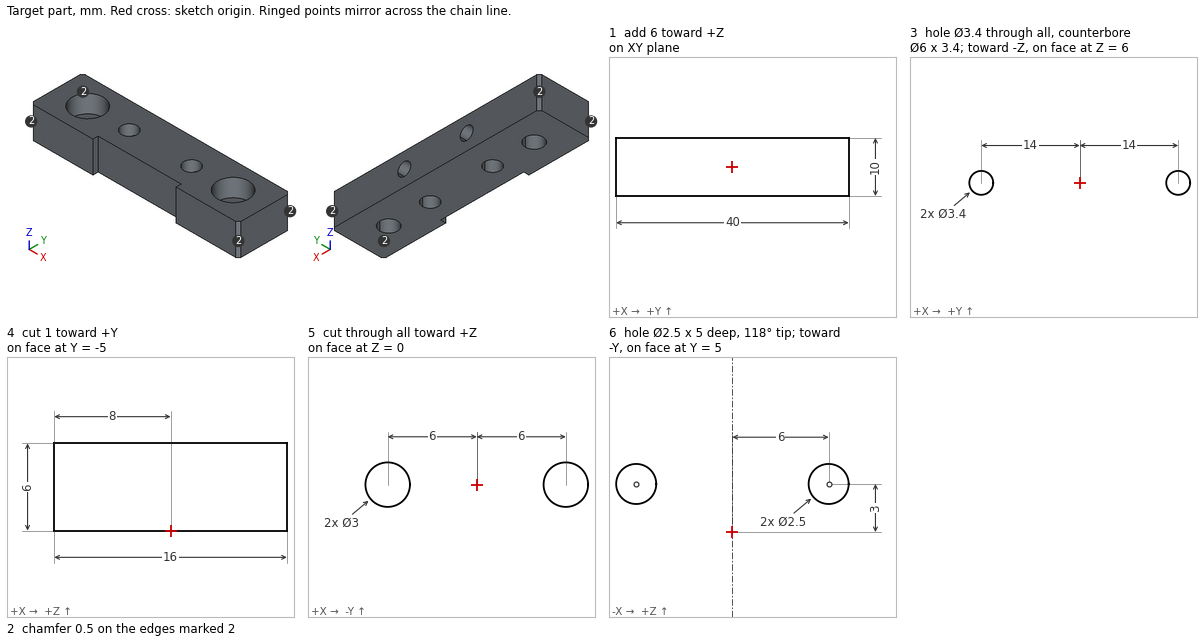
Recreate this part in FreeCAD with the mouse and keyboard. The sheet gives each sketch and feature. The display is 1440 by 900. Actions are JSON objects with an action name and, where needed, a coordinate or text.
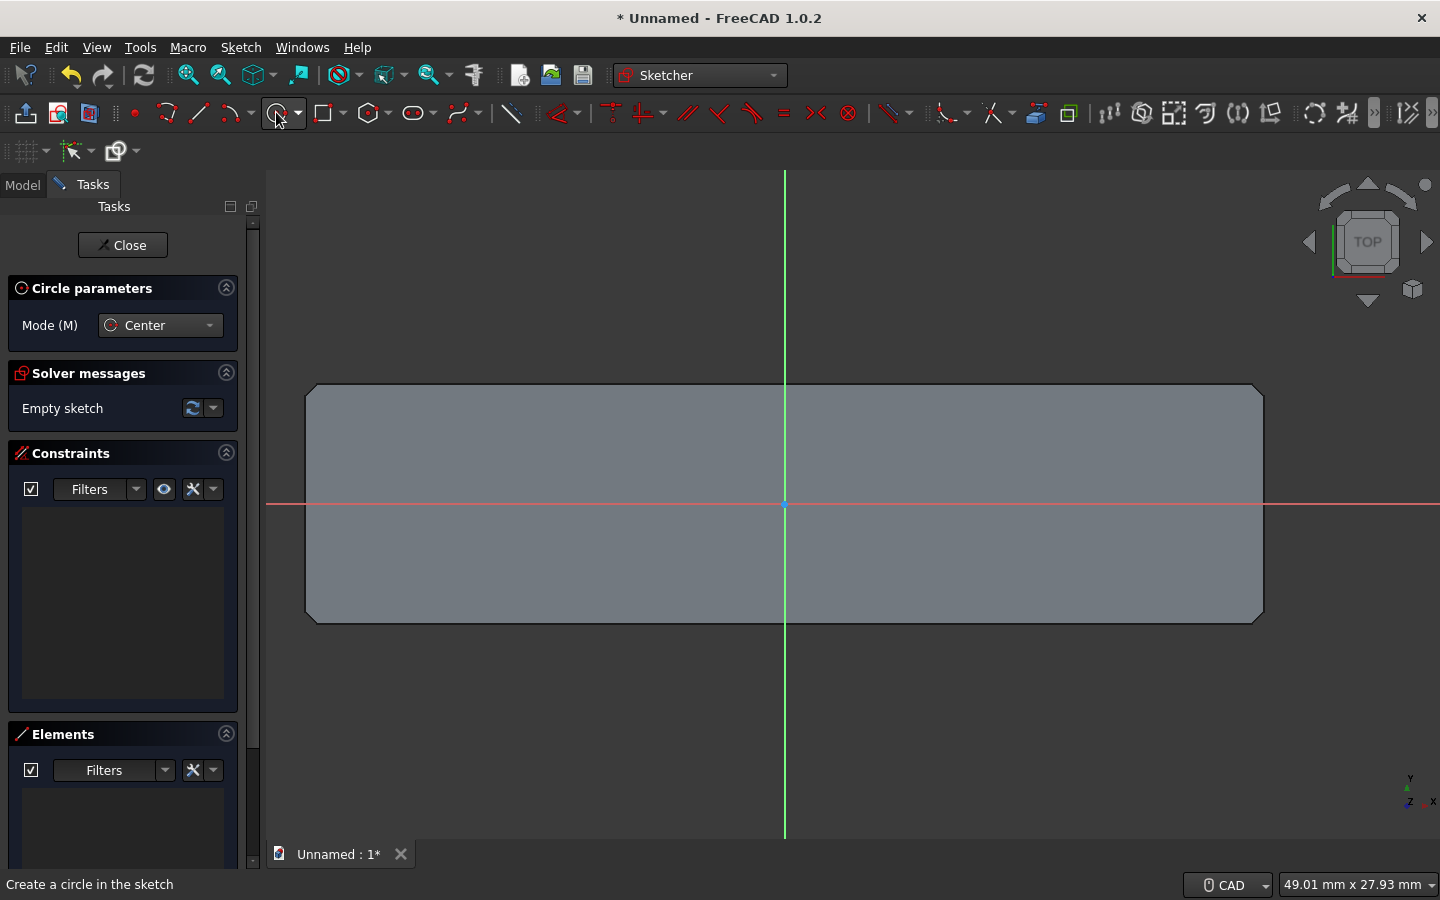
{"action": "left_click", "coordinate": [449, 504]}
{"action": "mouse_move", "coordinate": [478, 475]}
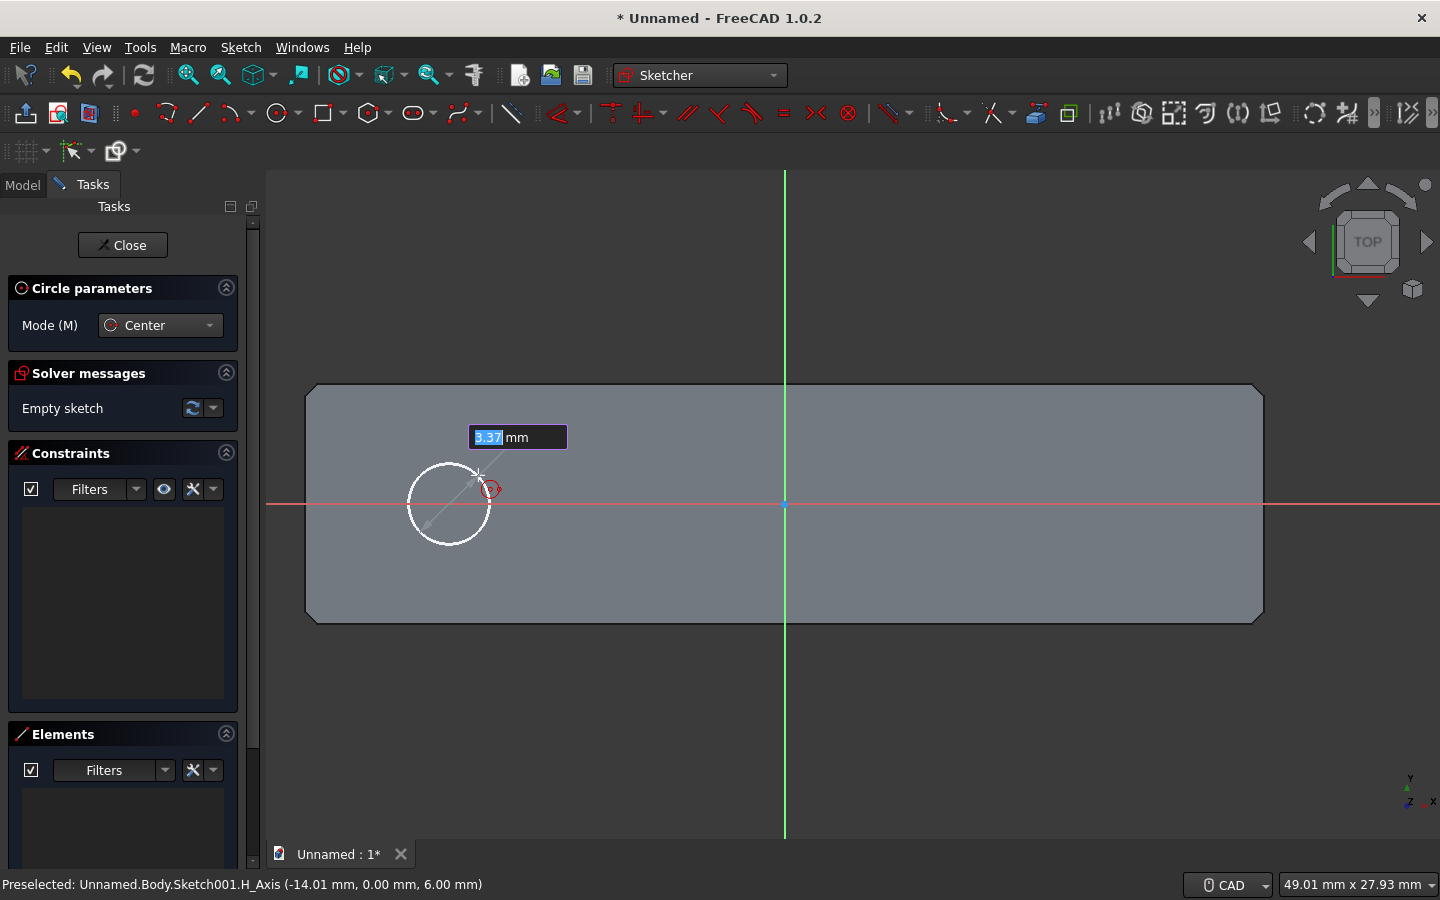
{"action": "type", "text": "3.4"}
{"action": "key", "text": "Return"}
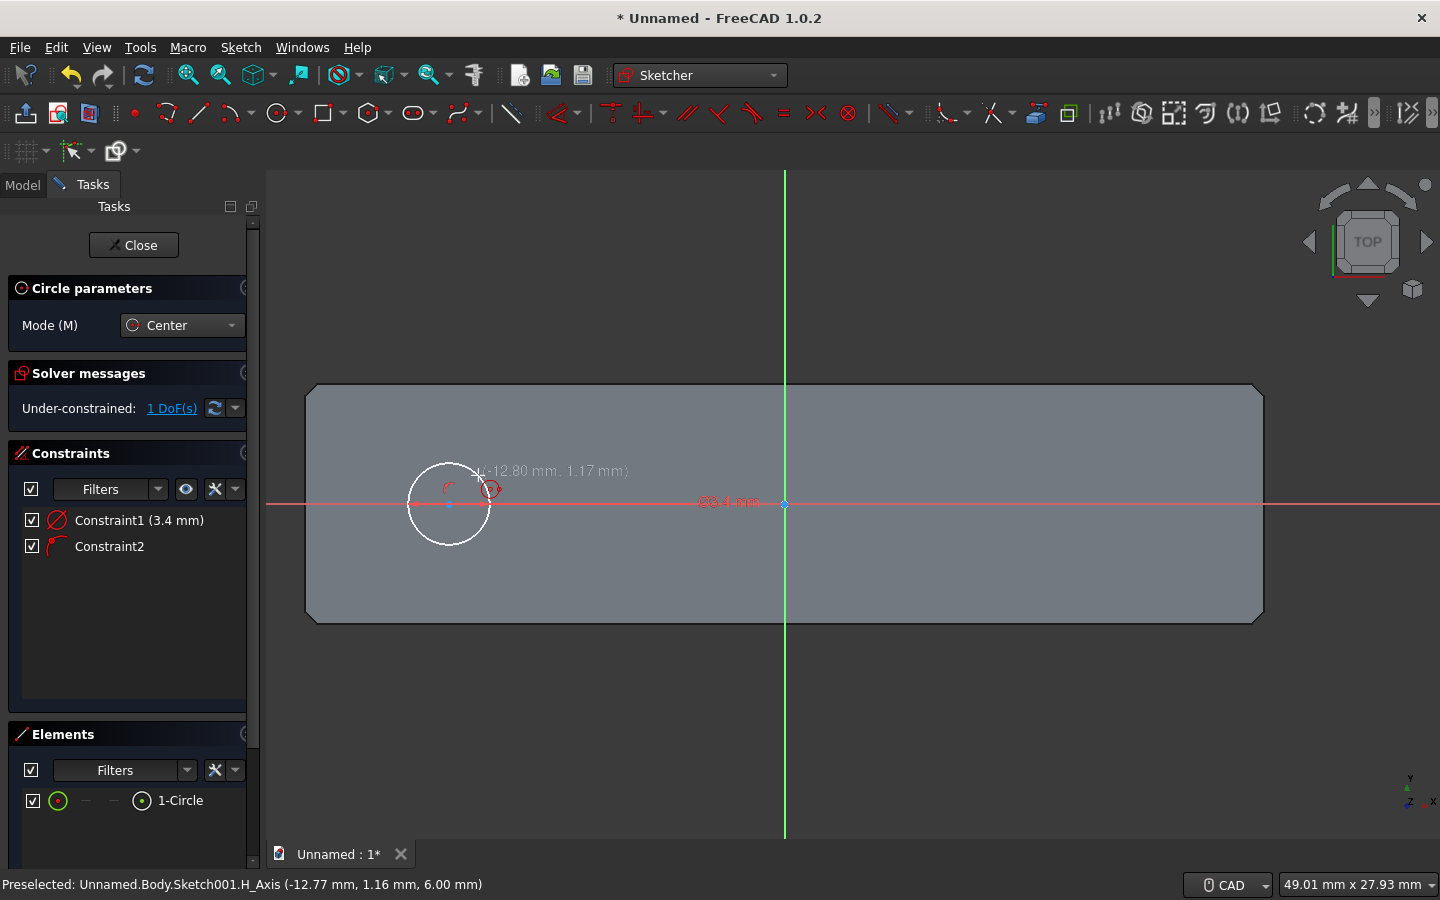
{"action": "left_click", "coordinate": [1120, 504]}
{"action": "mouse_move", "coordinate": [1149, 475]}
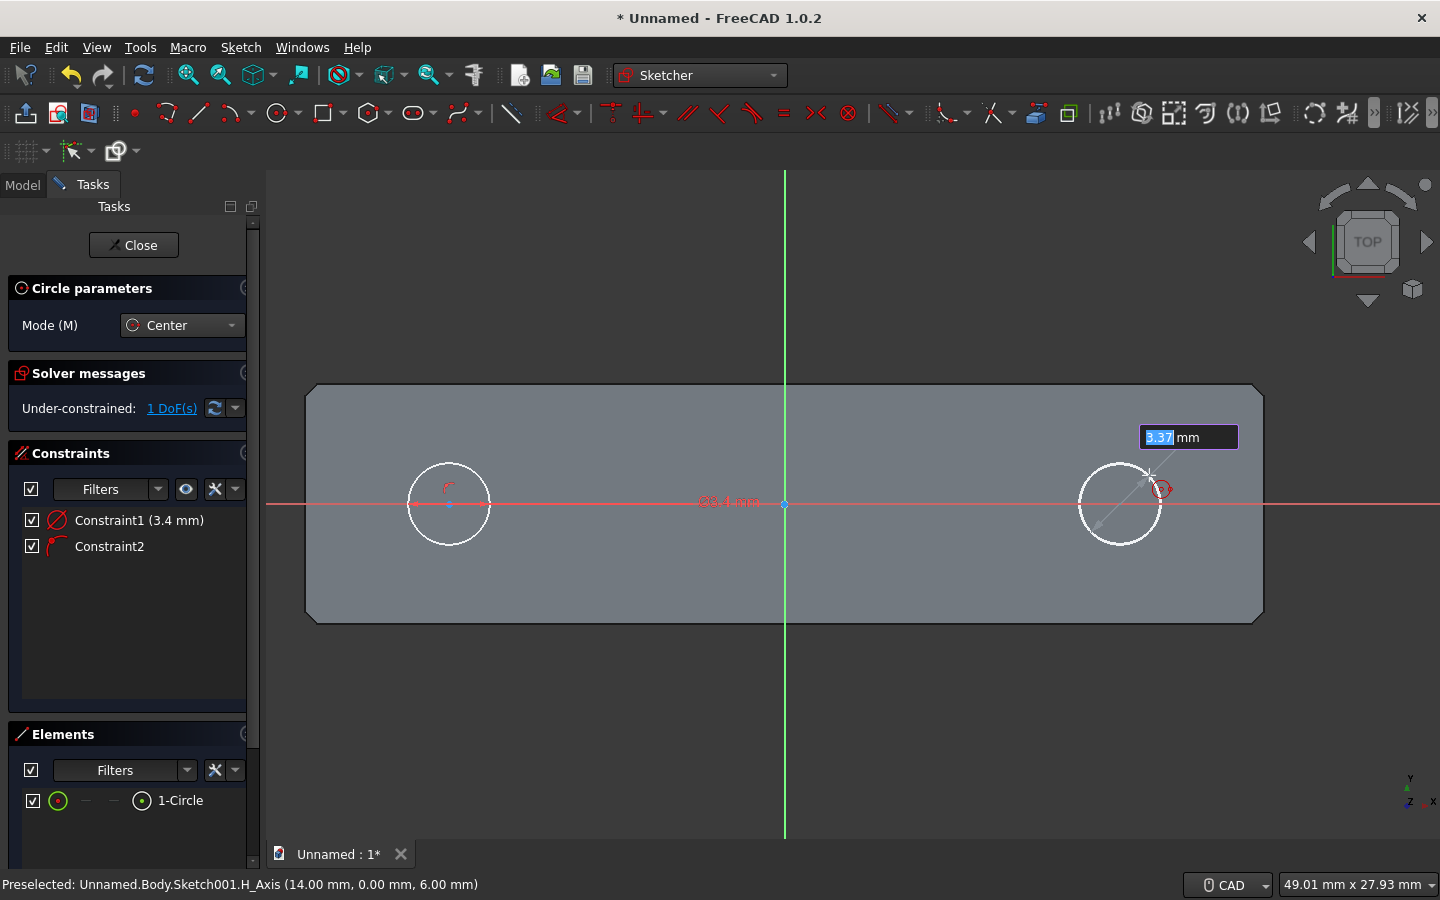
{"action": "type", "text": "3.4"}
{"action": "key", "text": "Return"}
{"action": "key", "text": "Escape"}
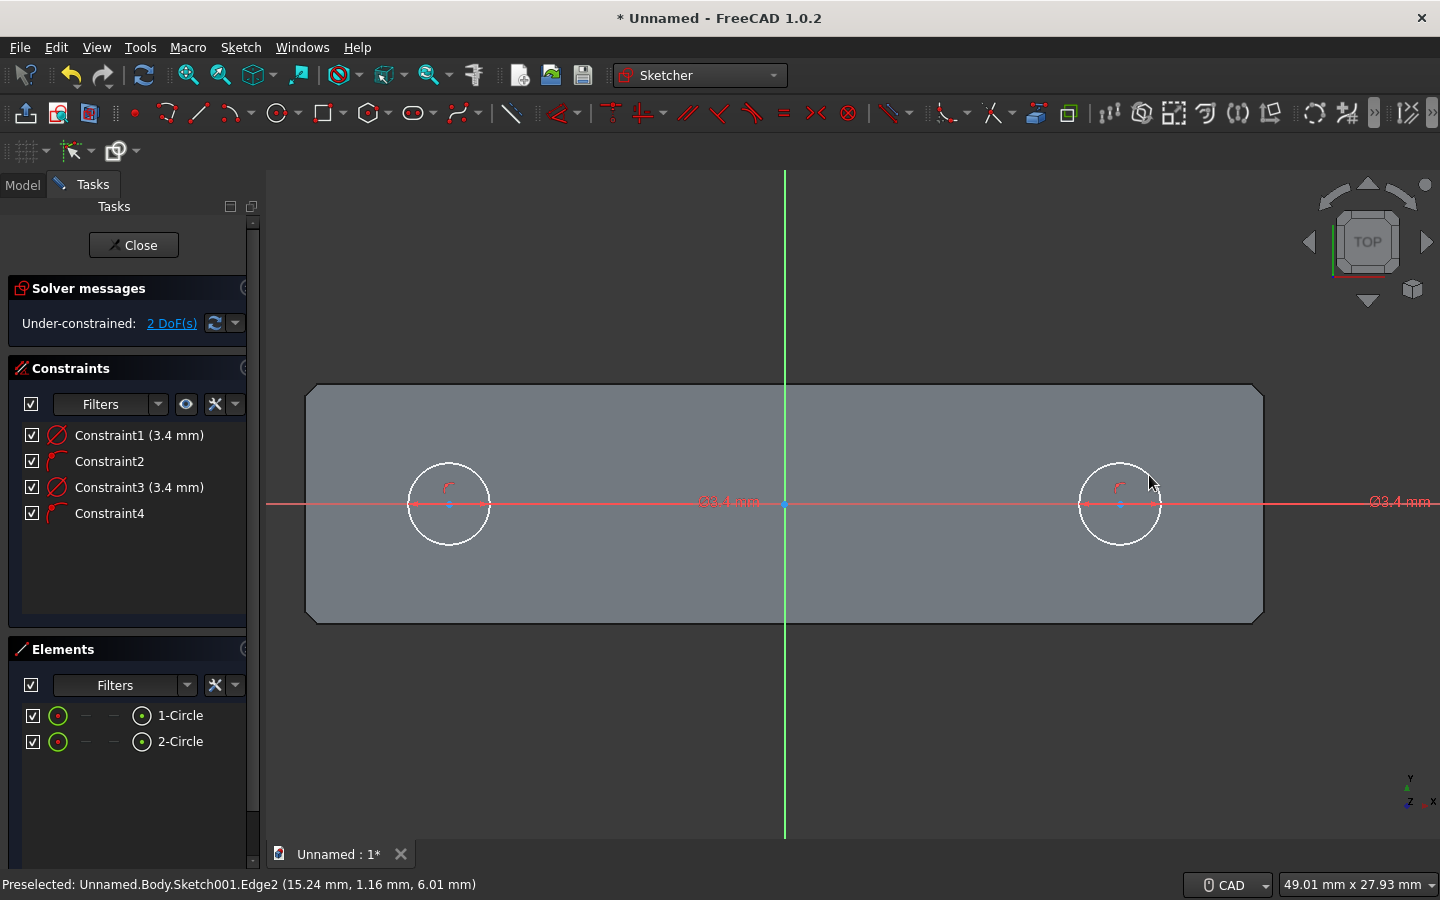
{"action": "left_click", "coordinate": [449, 504]}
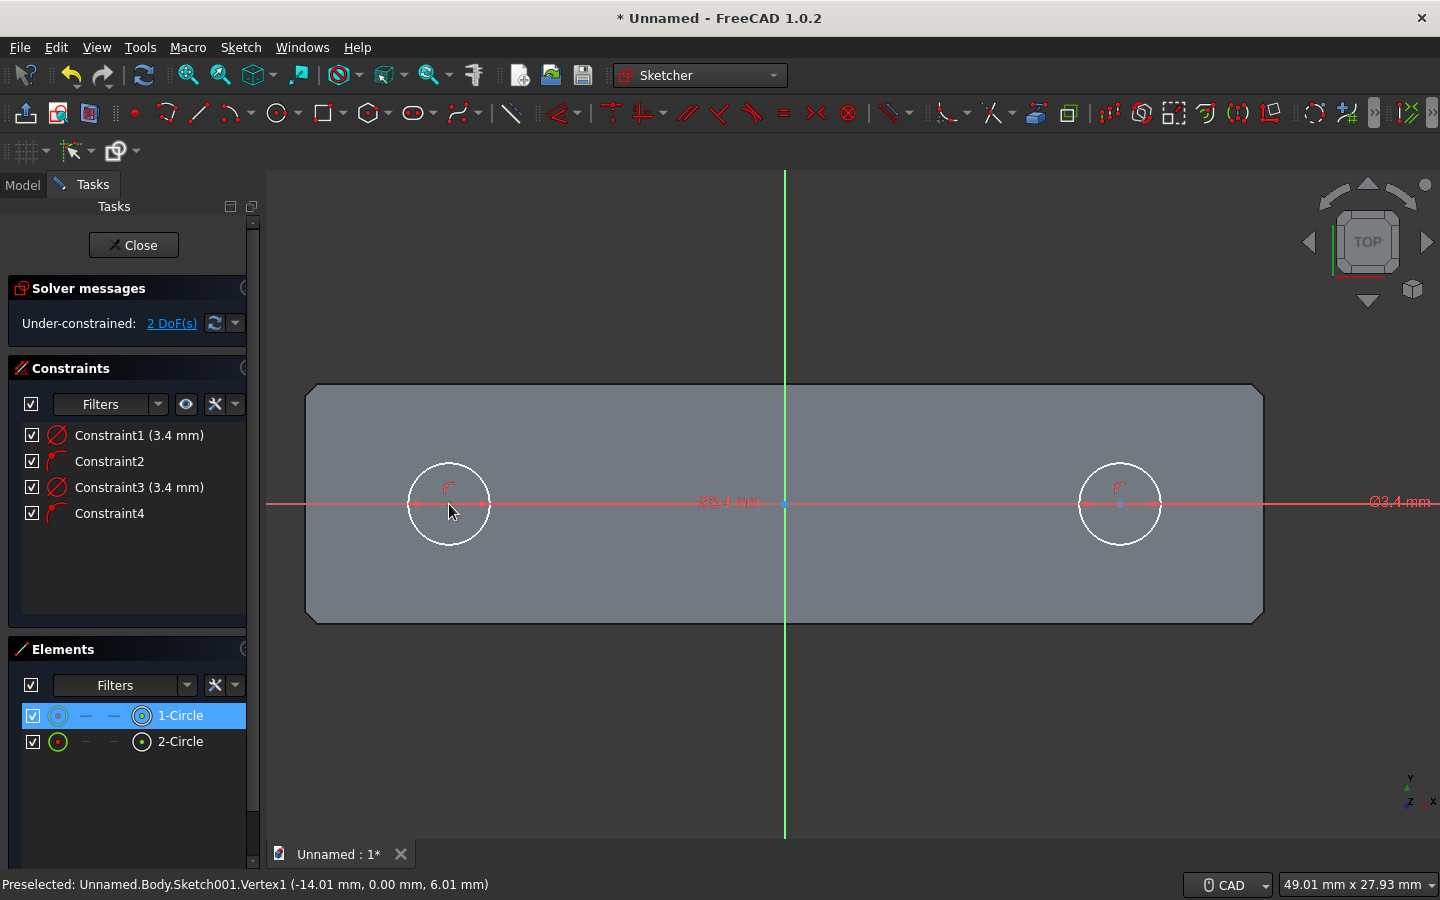
{"action": "left_click", "coordinate": [580, 114]}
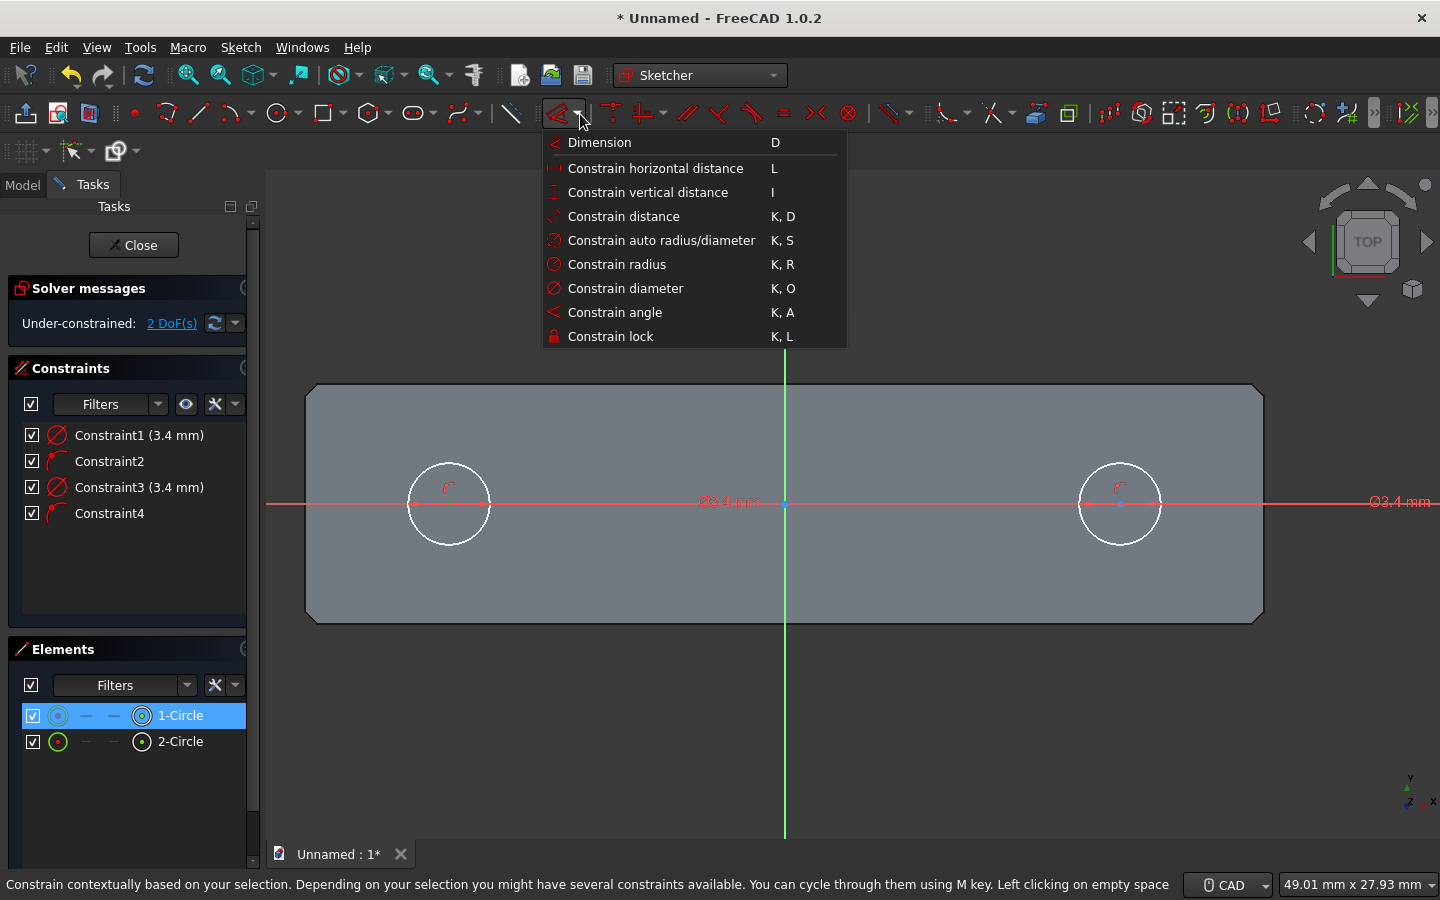
{"action": "left_click", "coordinate": [695, 168]}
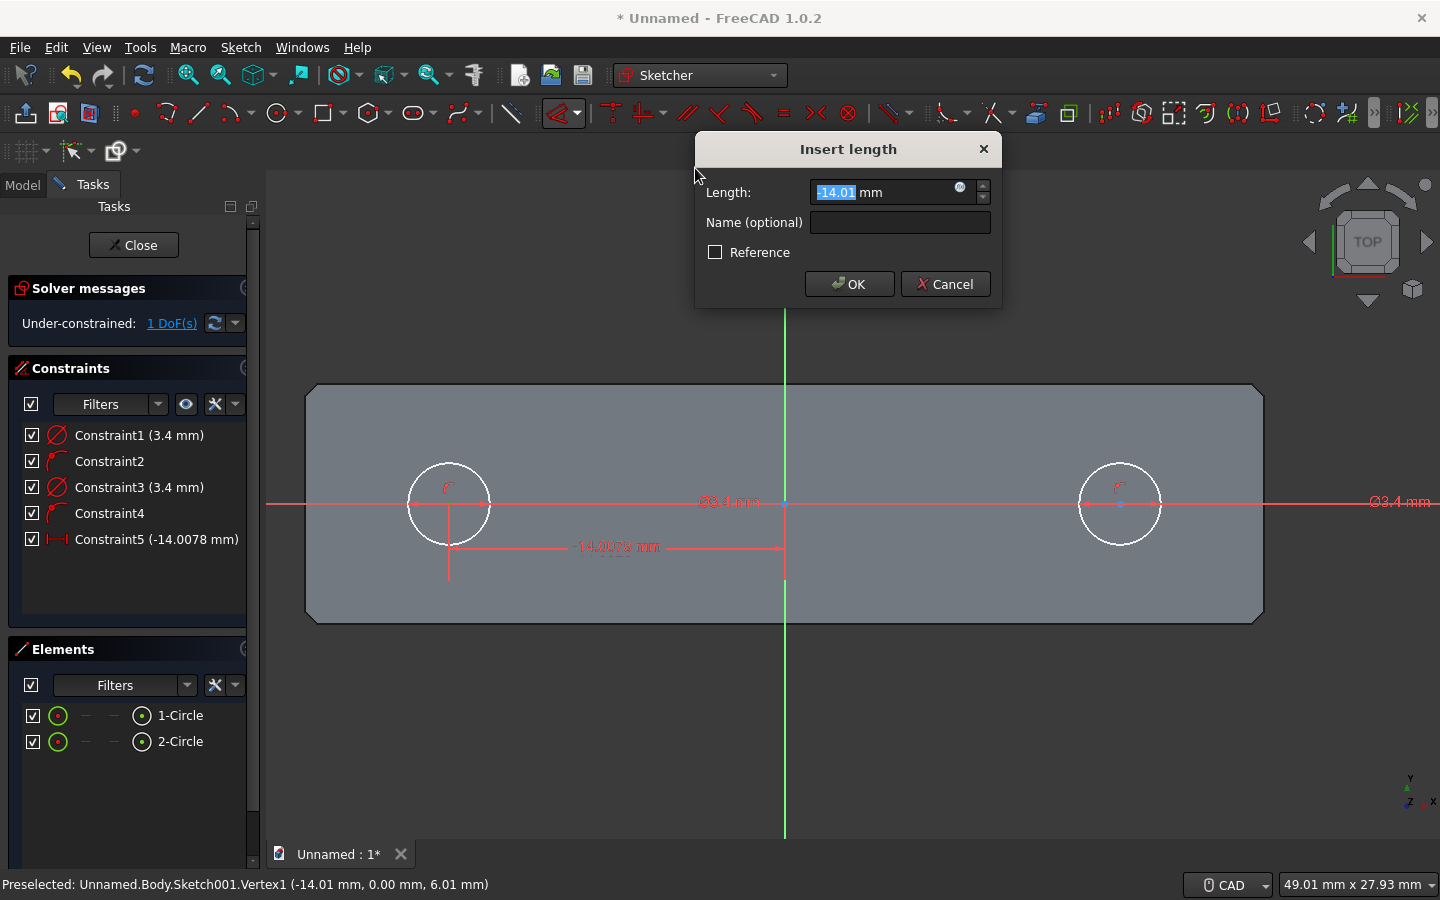
{"action": "type", "text": "-14"}
{"action": "key", "text": "Return"}